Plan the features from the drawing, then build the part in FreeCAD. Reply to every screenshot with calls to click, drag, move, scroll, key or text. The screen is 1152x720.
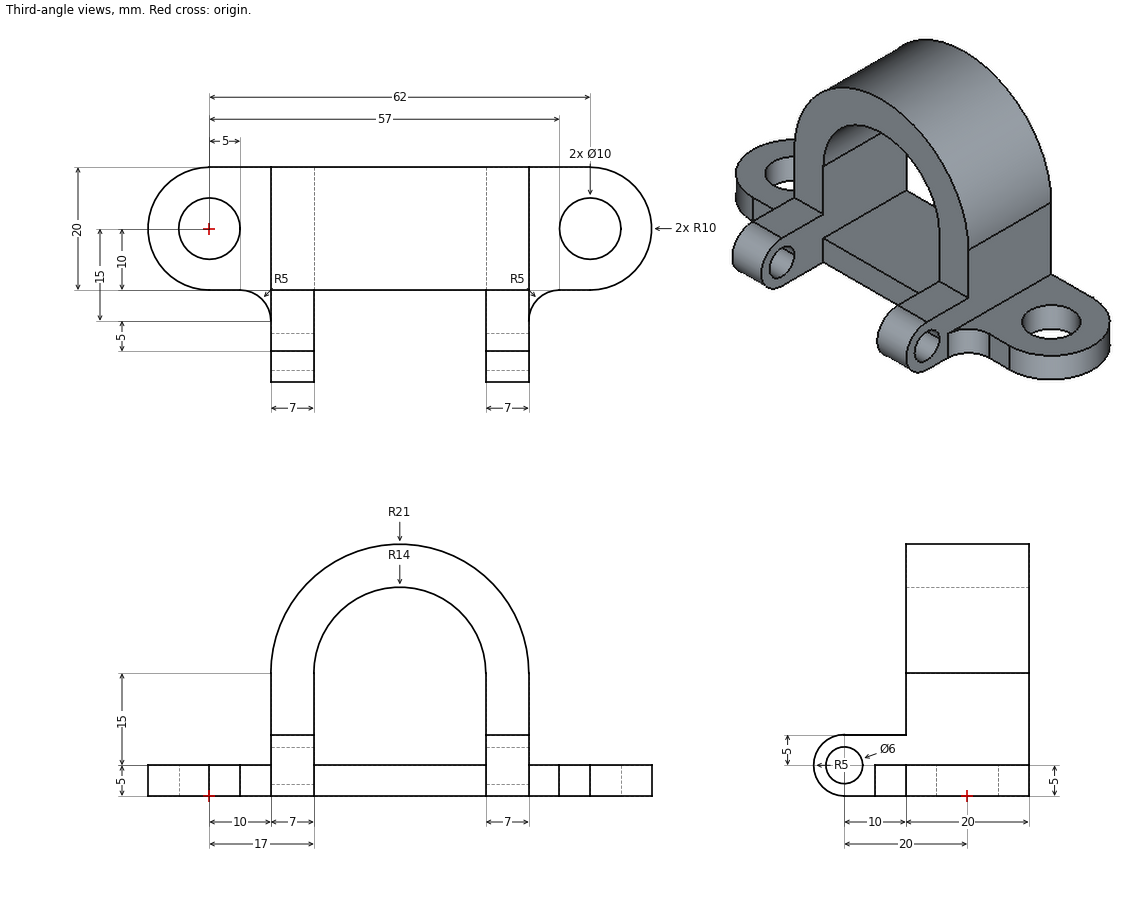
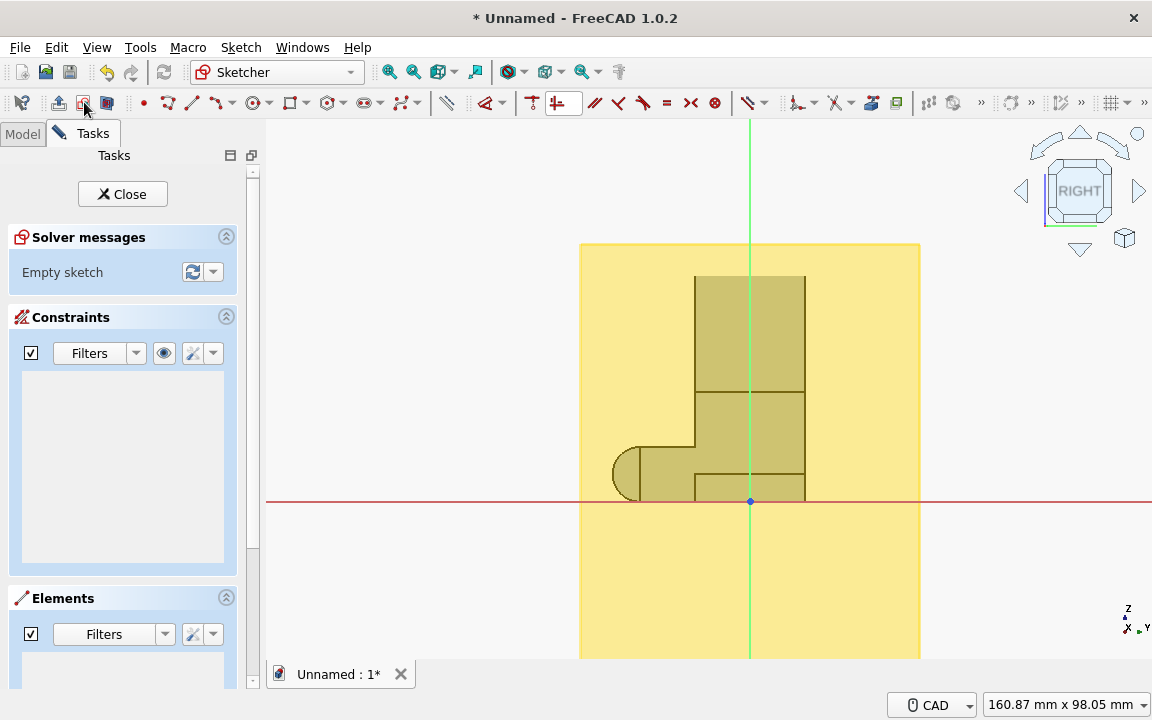
scroll(623, 491, up, 9)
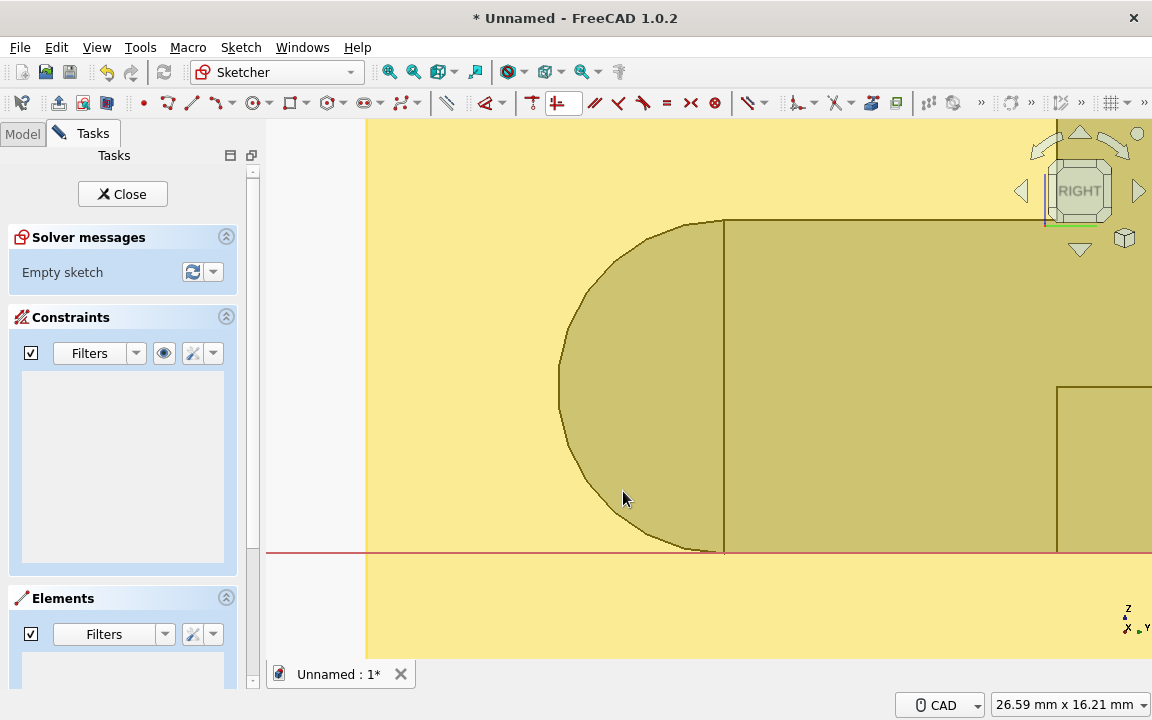
click(192, 104)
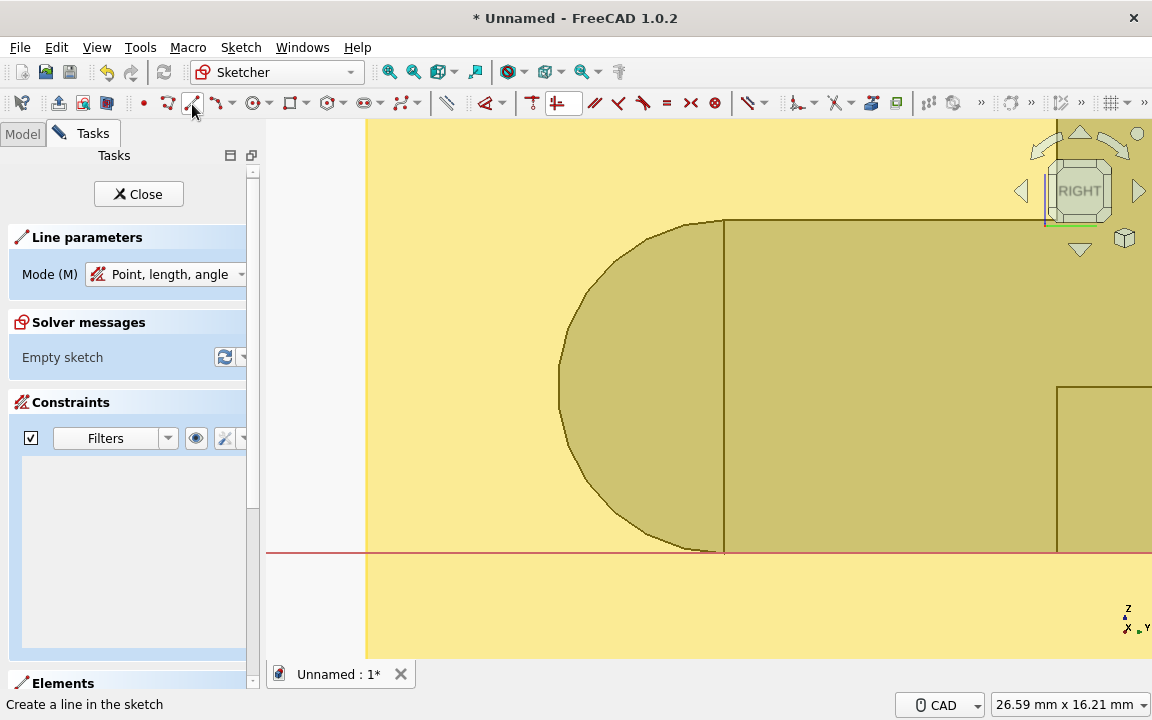
click(724, 553)
click(724, 220)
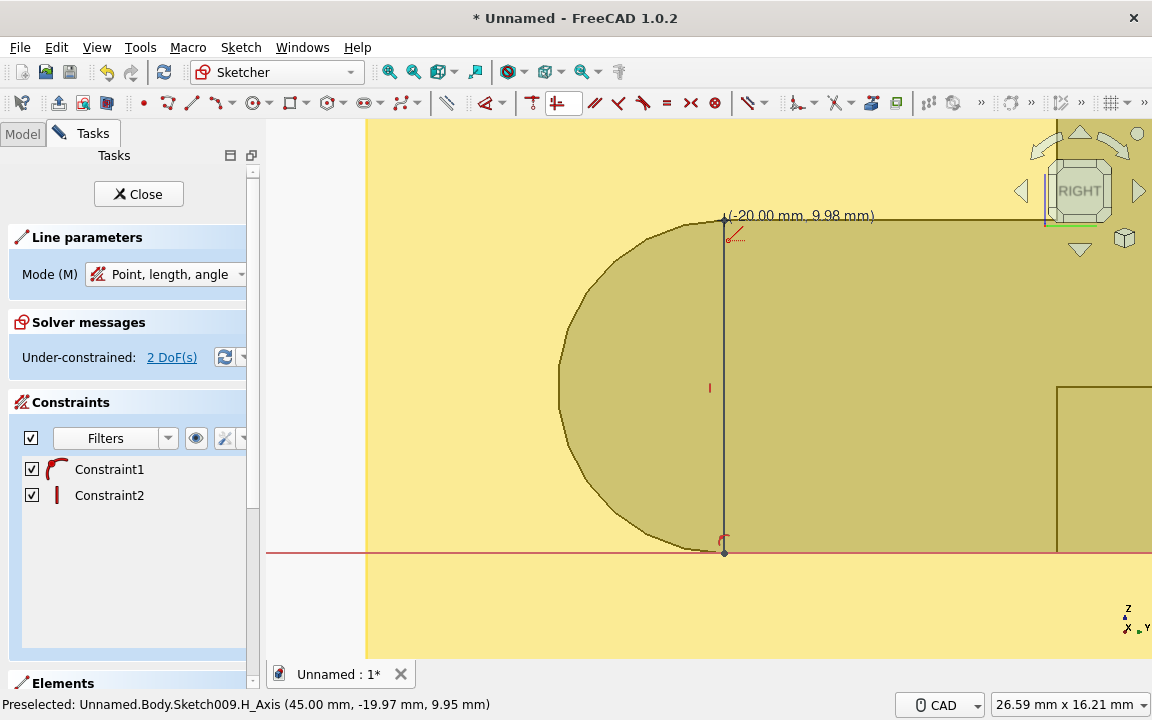
click(216, 104)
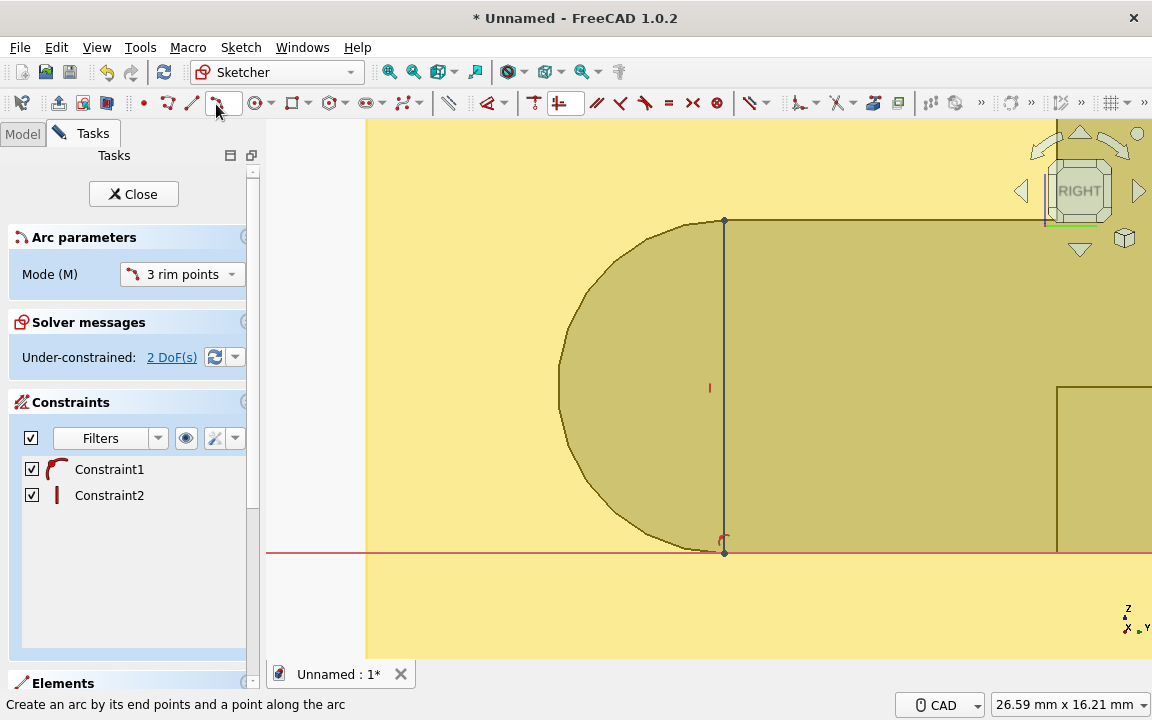
click(724, 221)
click(724, 553)
click(558, 387)
key(Escape)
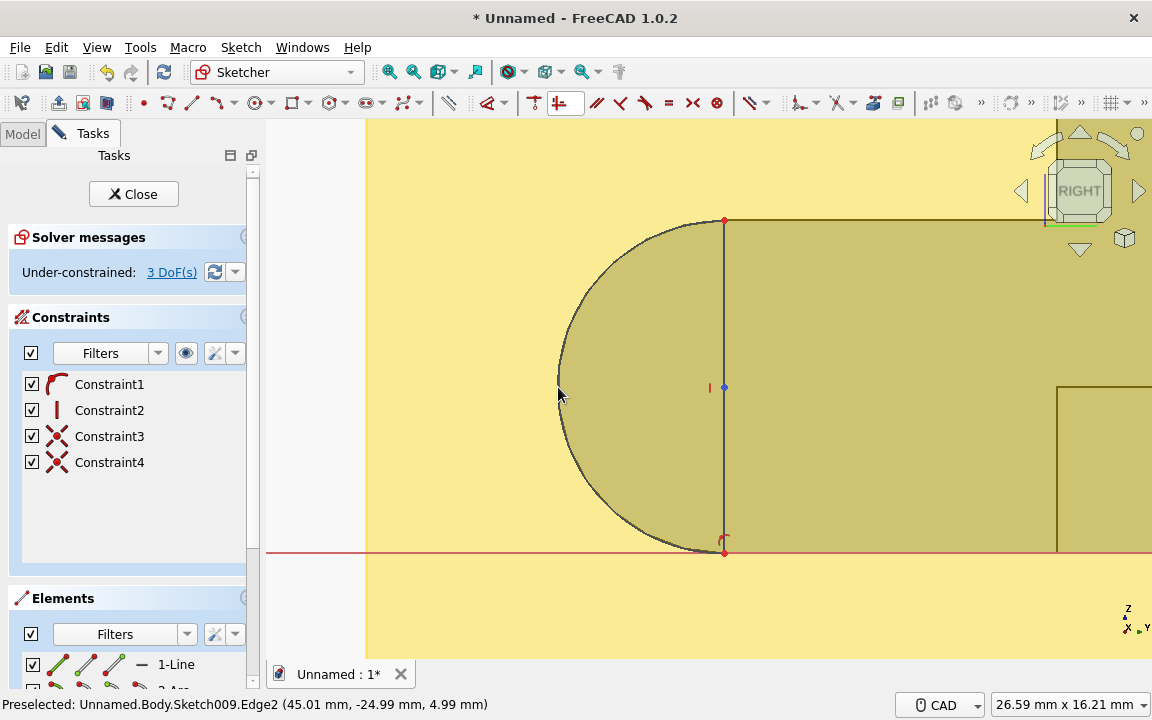
click(488, 104)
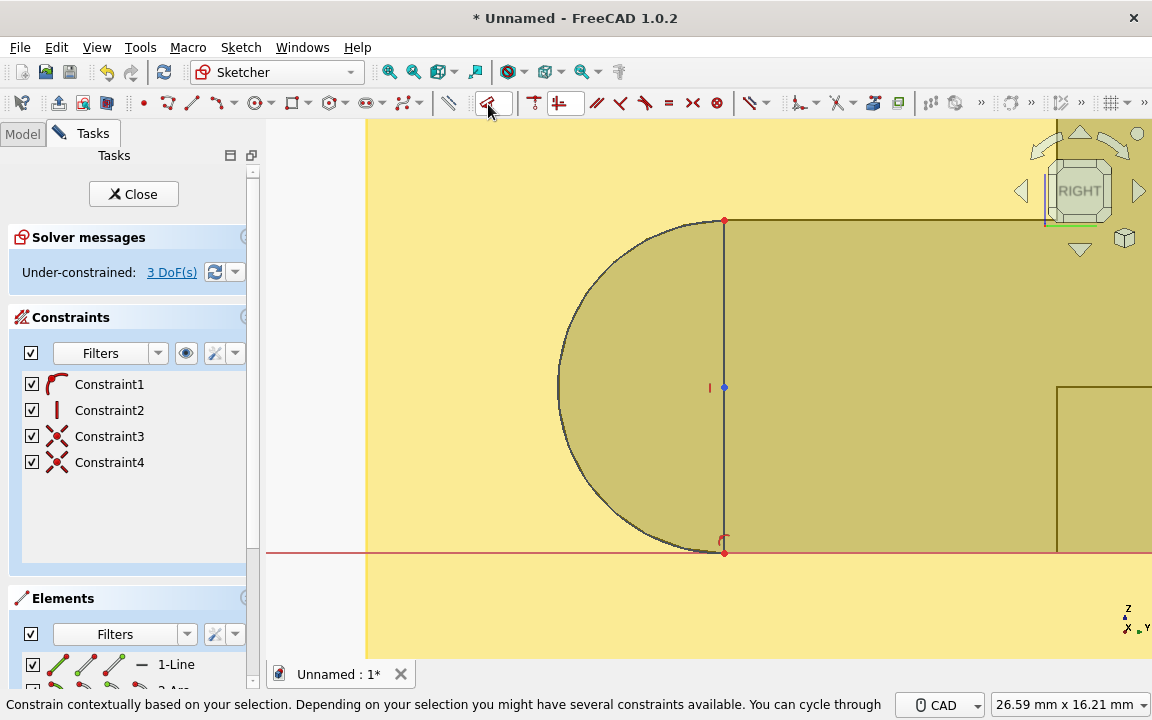
click(590, 290)
click(564, 271)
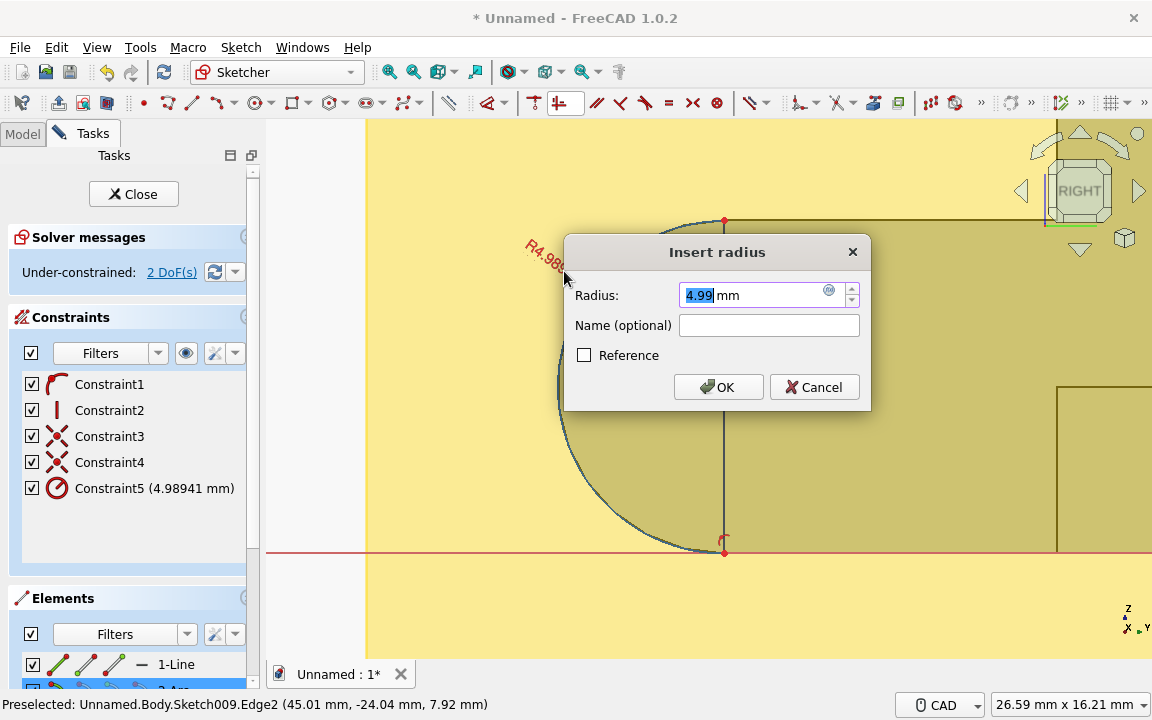
text(5)
key(Return)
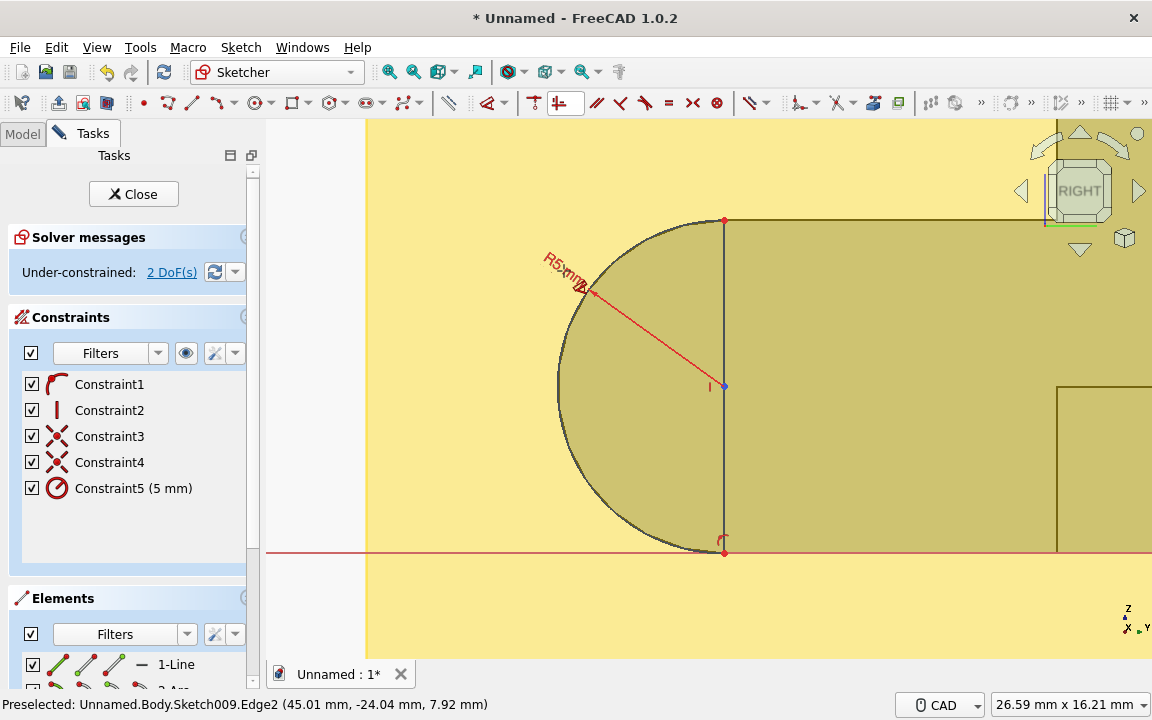
click(724, 553)
click(855, 587)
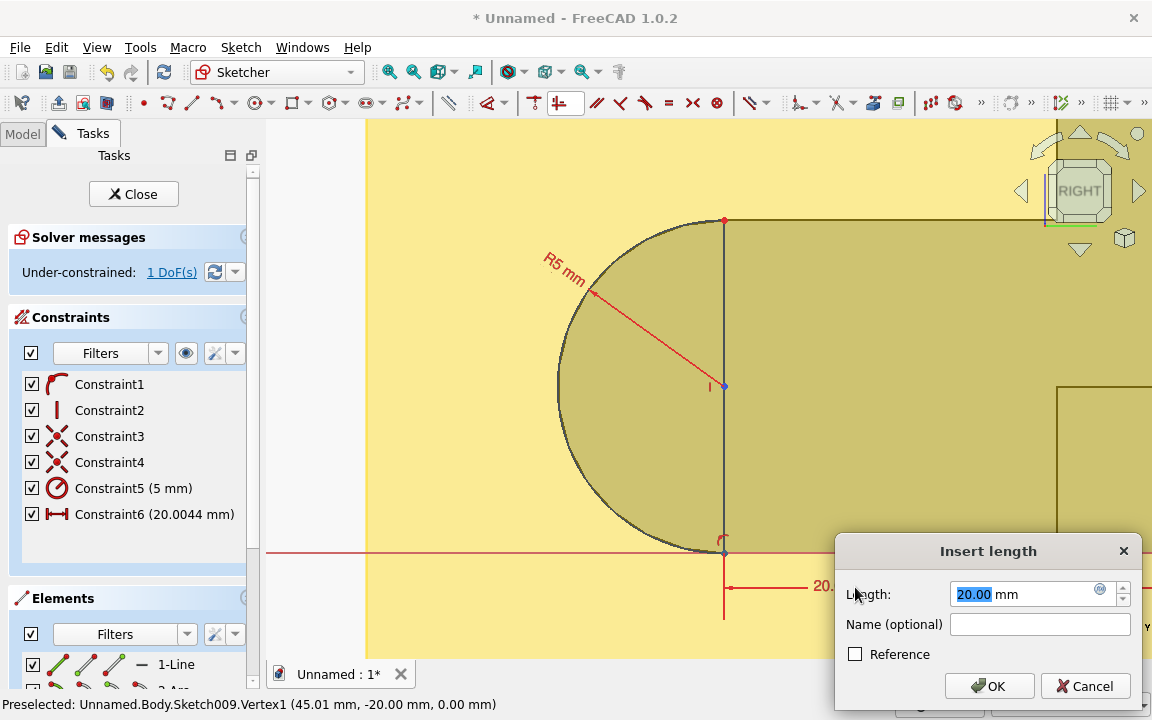
text(20)
key(Return)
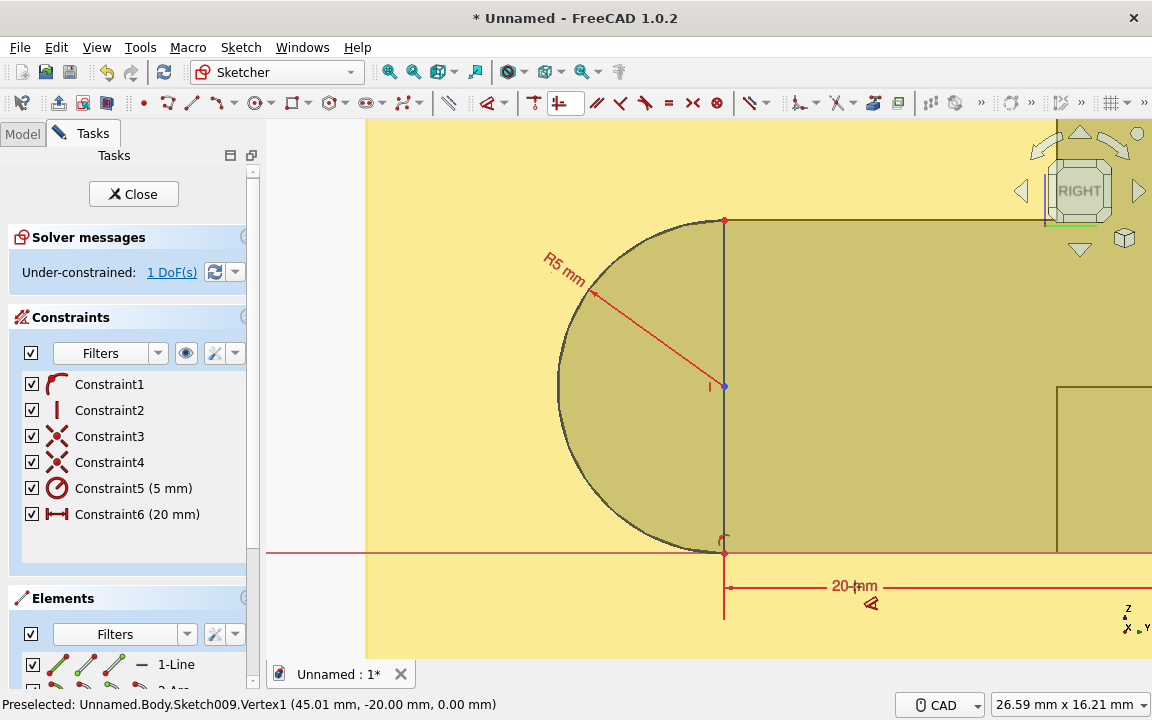
click(724, 387)
click(764, 587)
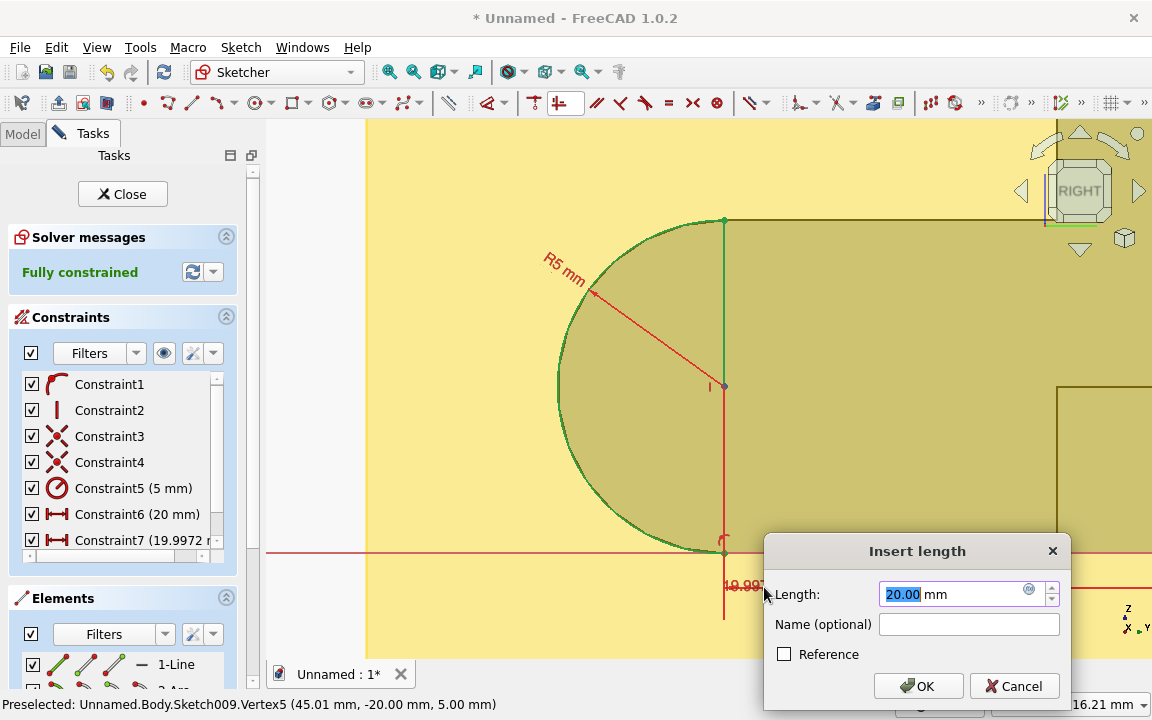
text(20)
key(Return)
key(Escape)